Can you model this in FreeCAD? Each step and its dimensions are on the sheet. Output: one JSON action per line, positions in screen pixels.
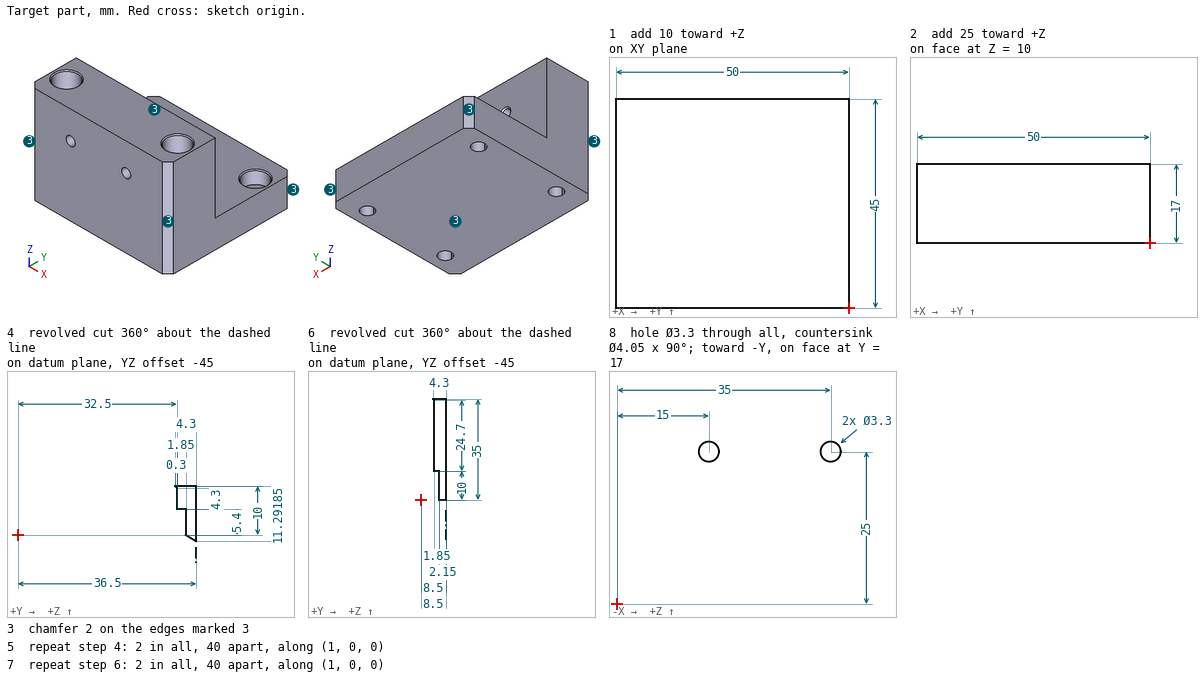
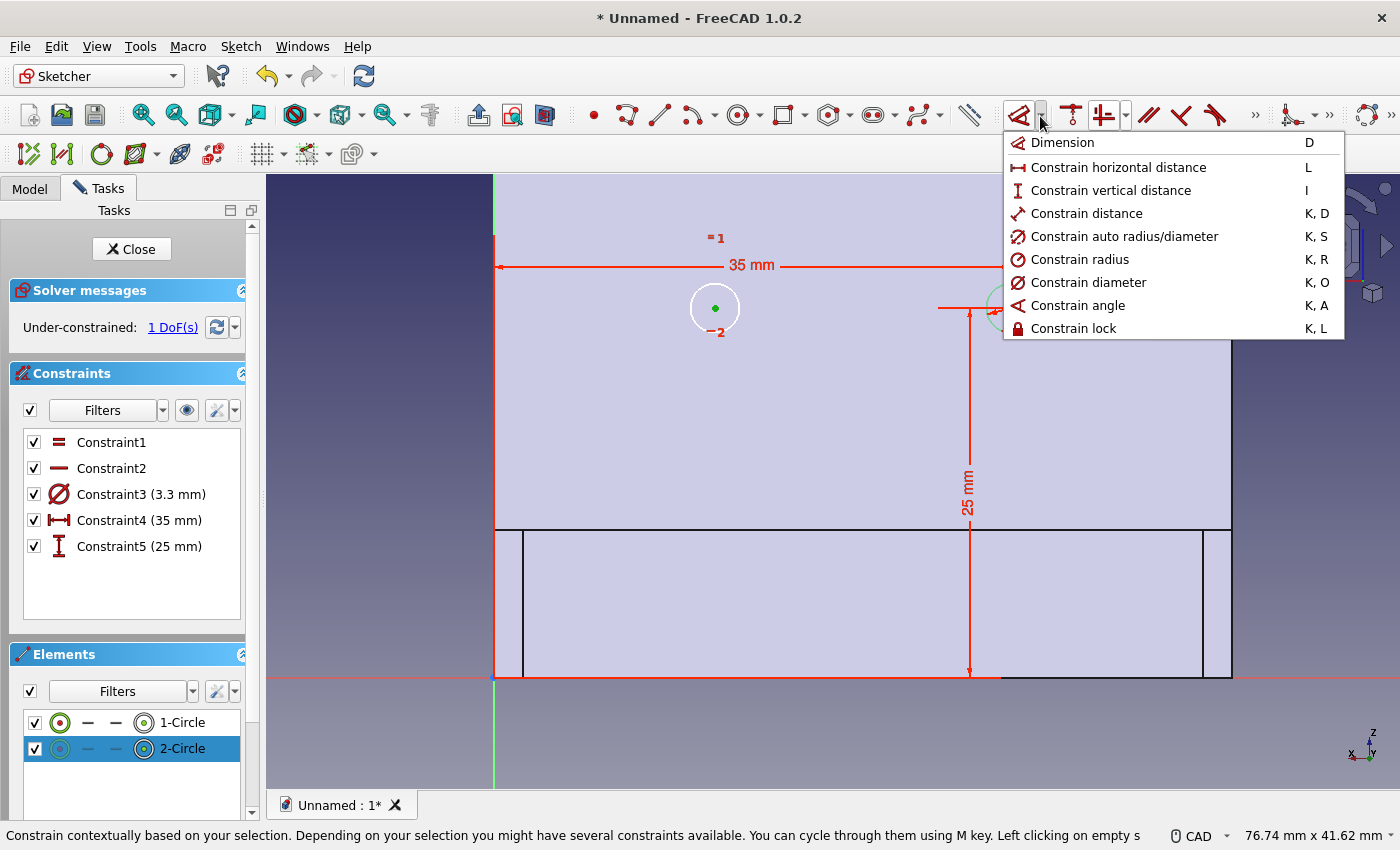
{"action": "left_click", "coordinate": [1174, 168]}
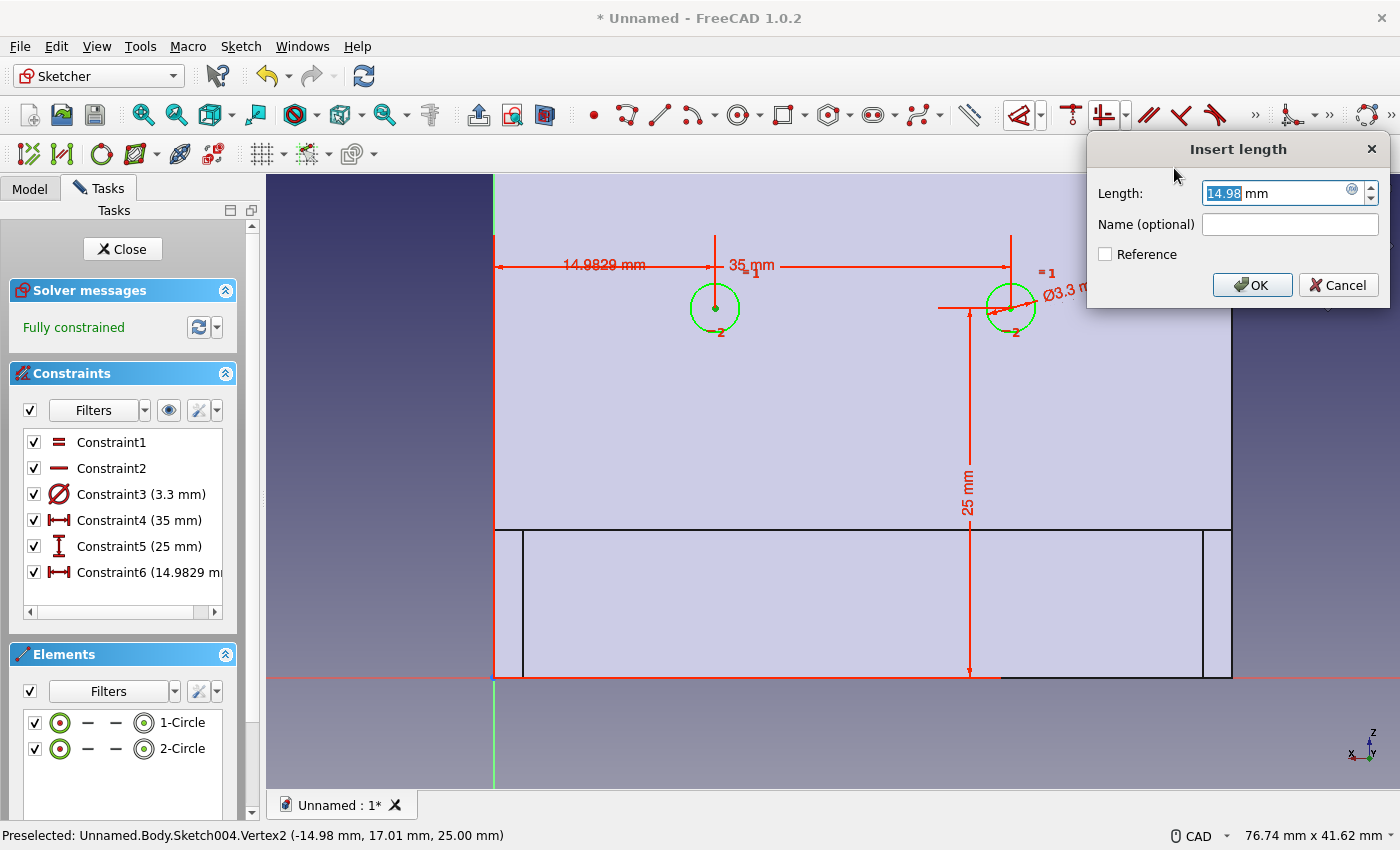
{"action": "type", "text": "15"}
{"action": "key", "text": "Return"}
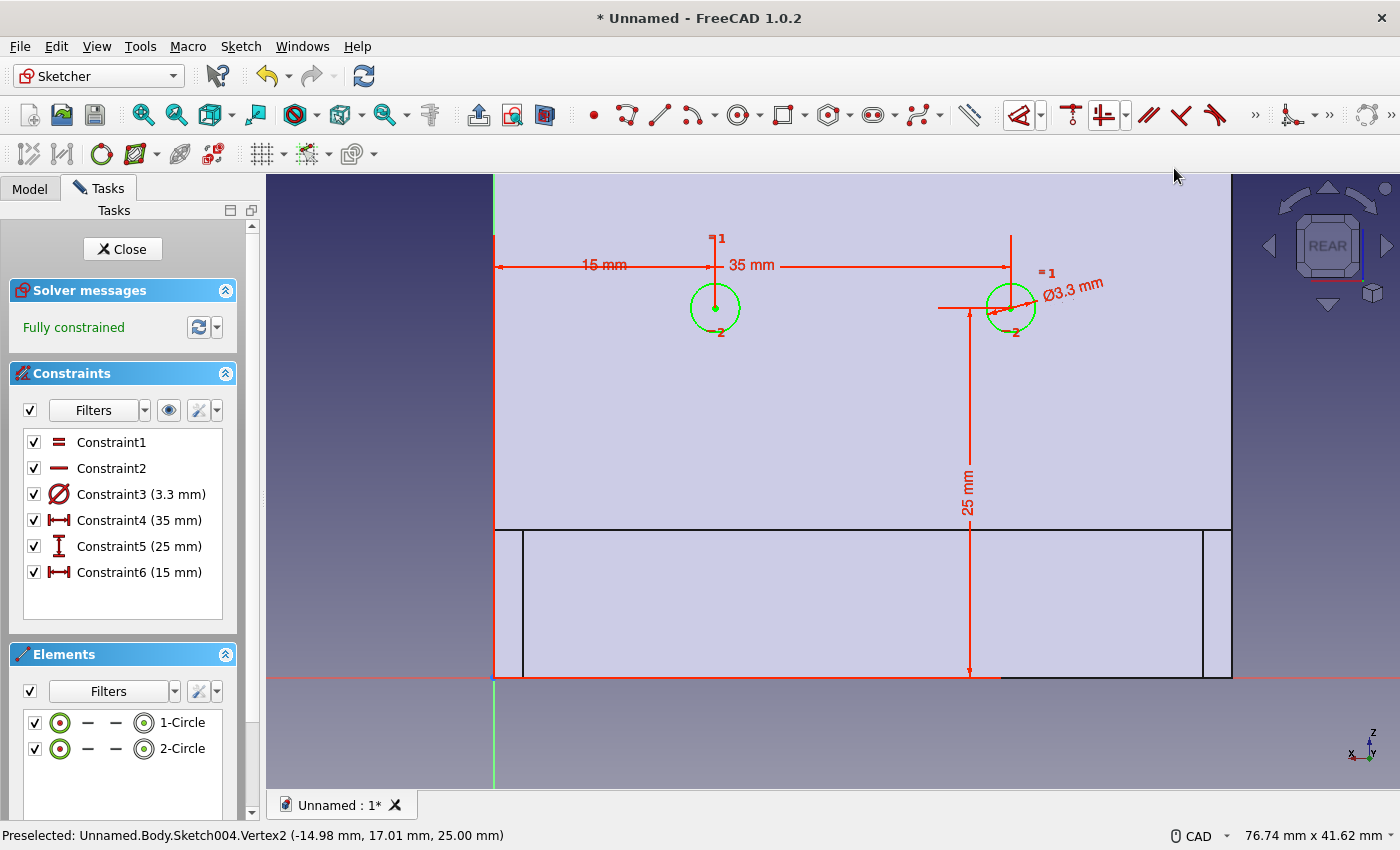
{"action": "left_click", "coordinate": [123, 249]}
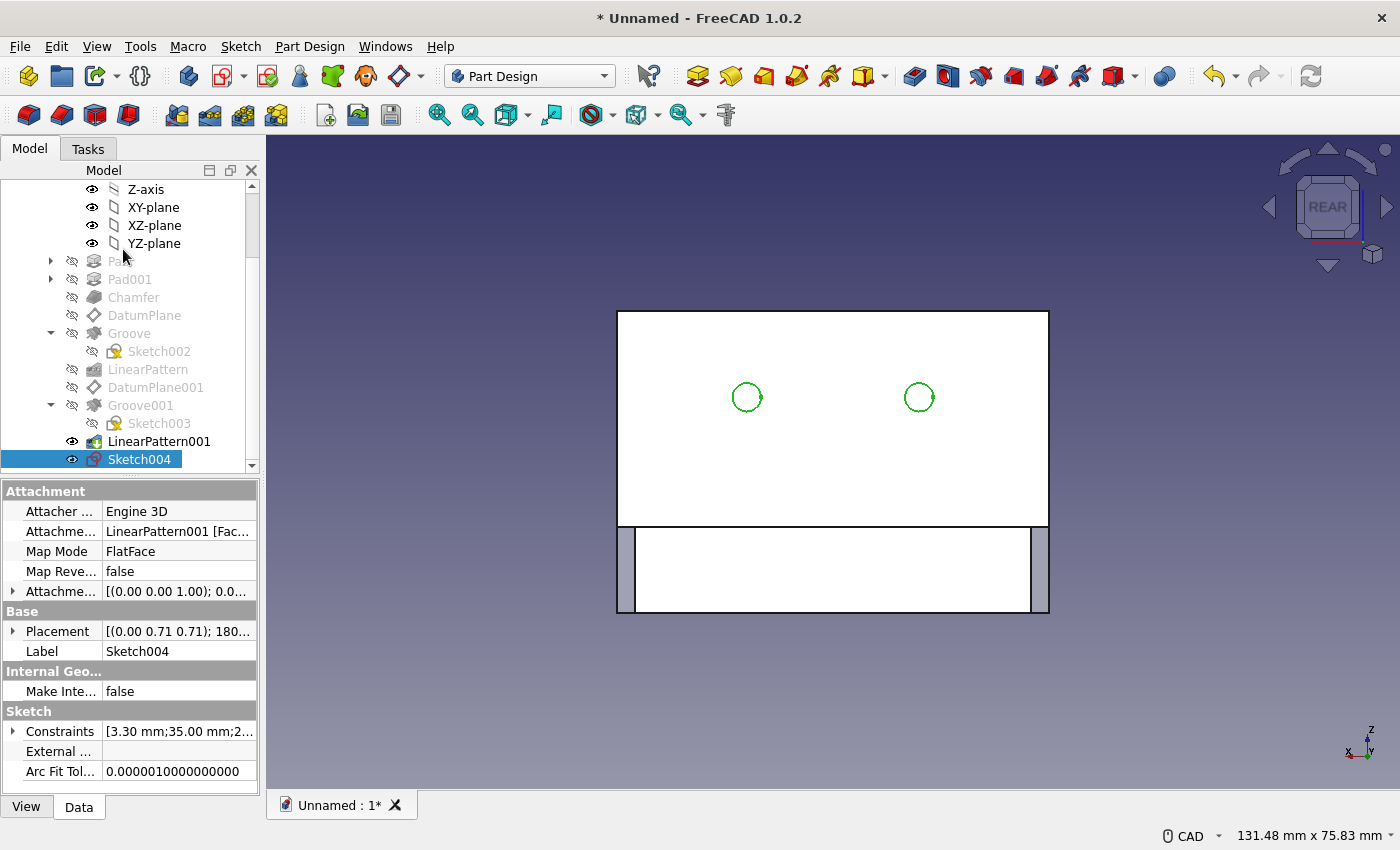
{"action": "left_click", "coordinate": [948, 76]}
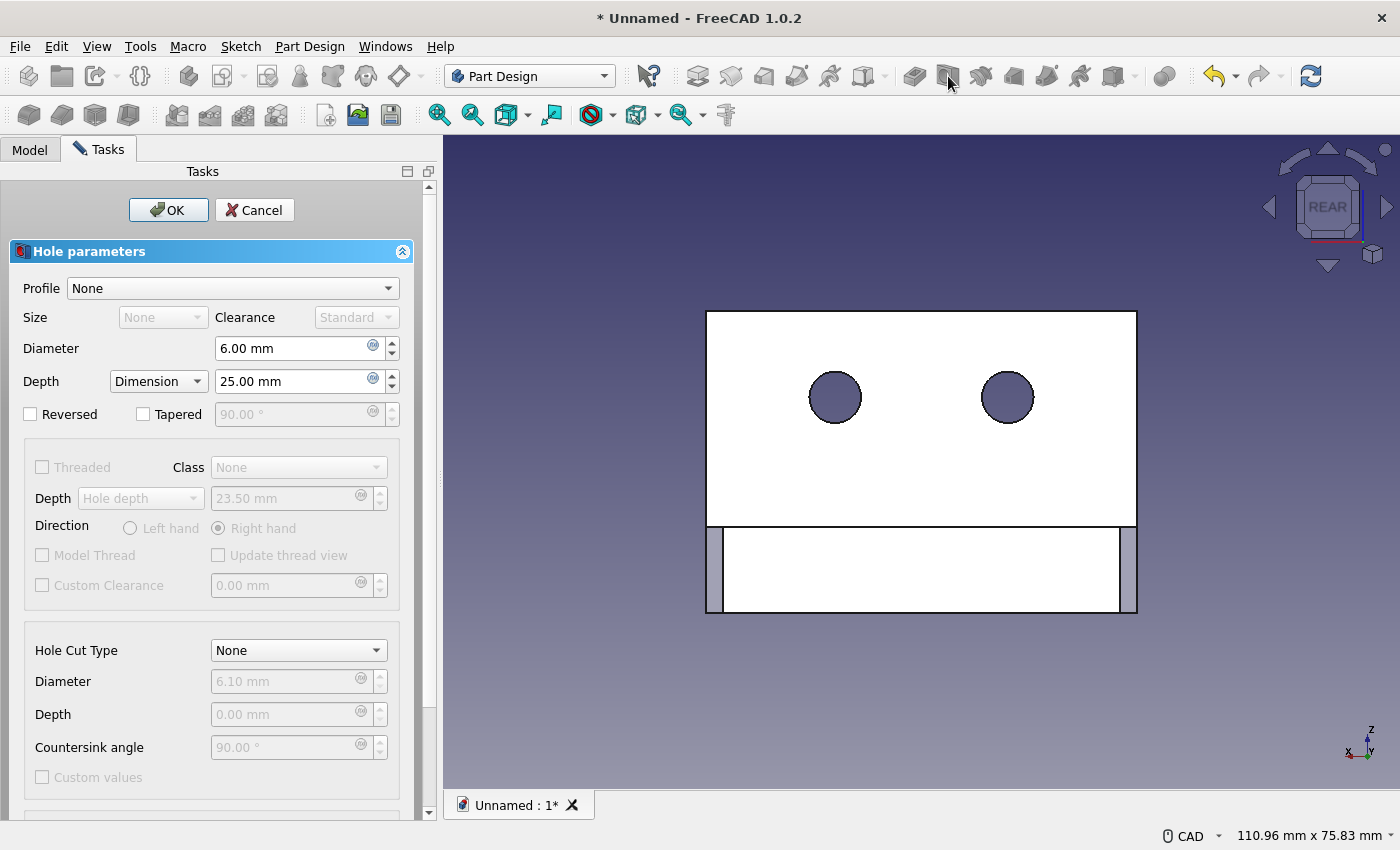
{"action": "triple_click", "coordinate": [300, 348]}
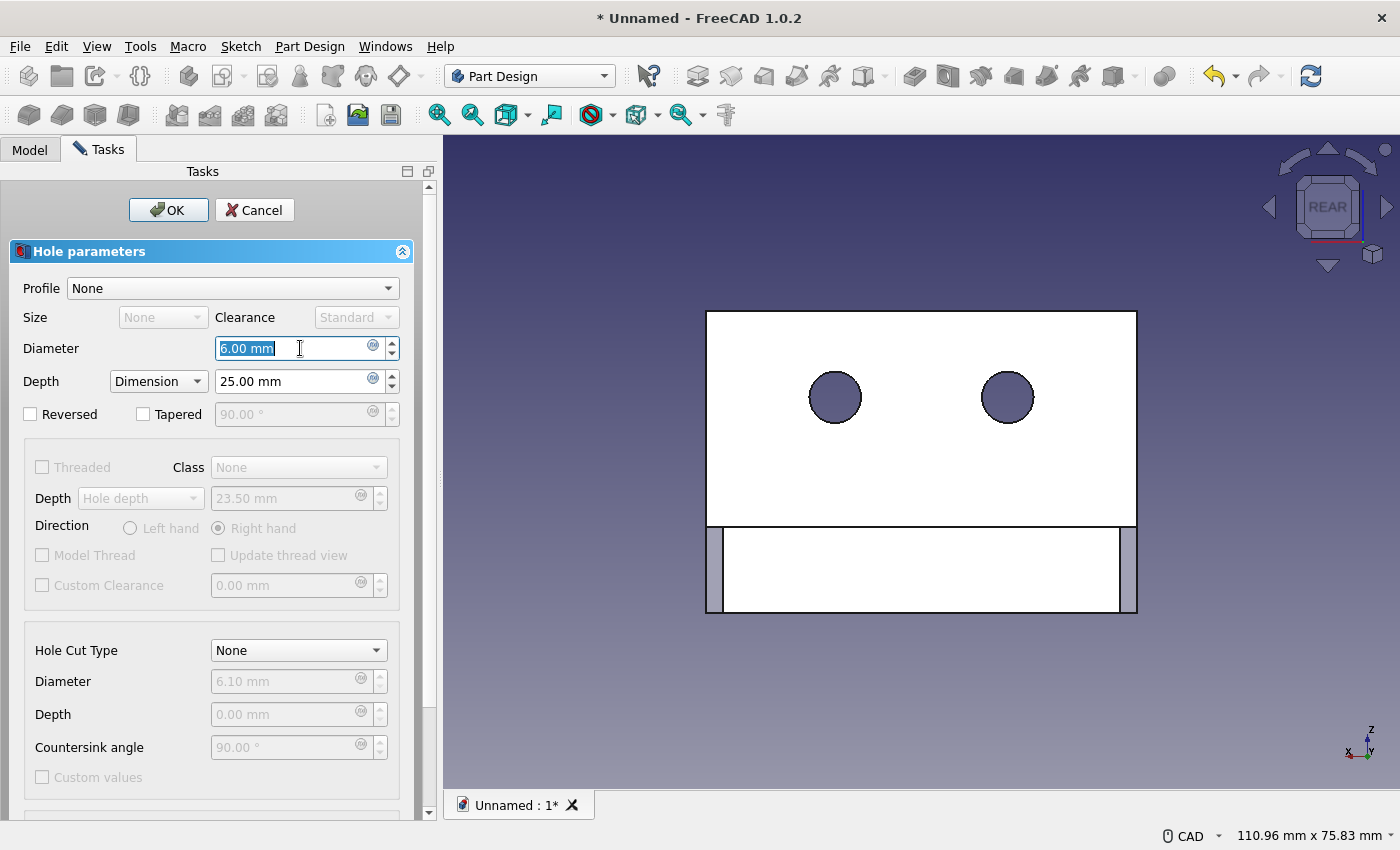
{"action": "type", "text": "3.3"}
{"action": "key", "text": "Tab"}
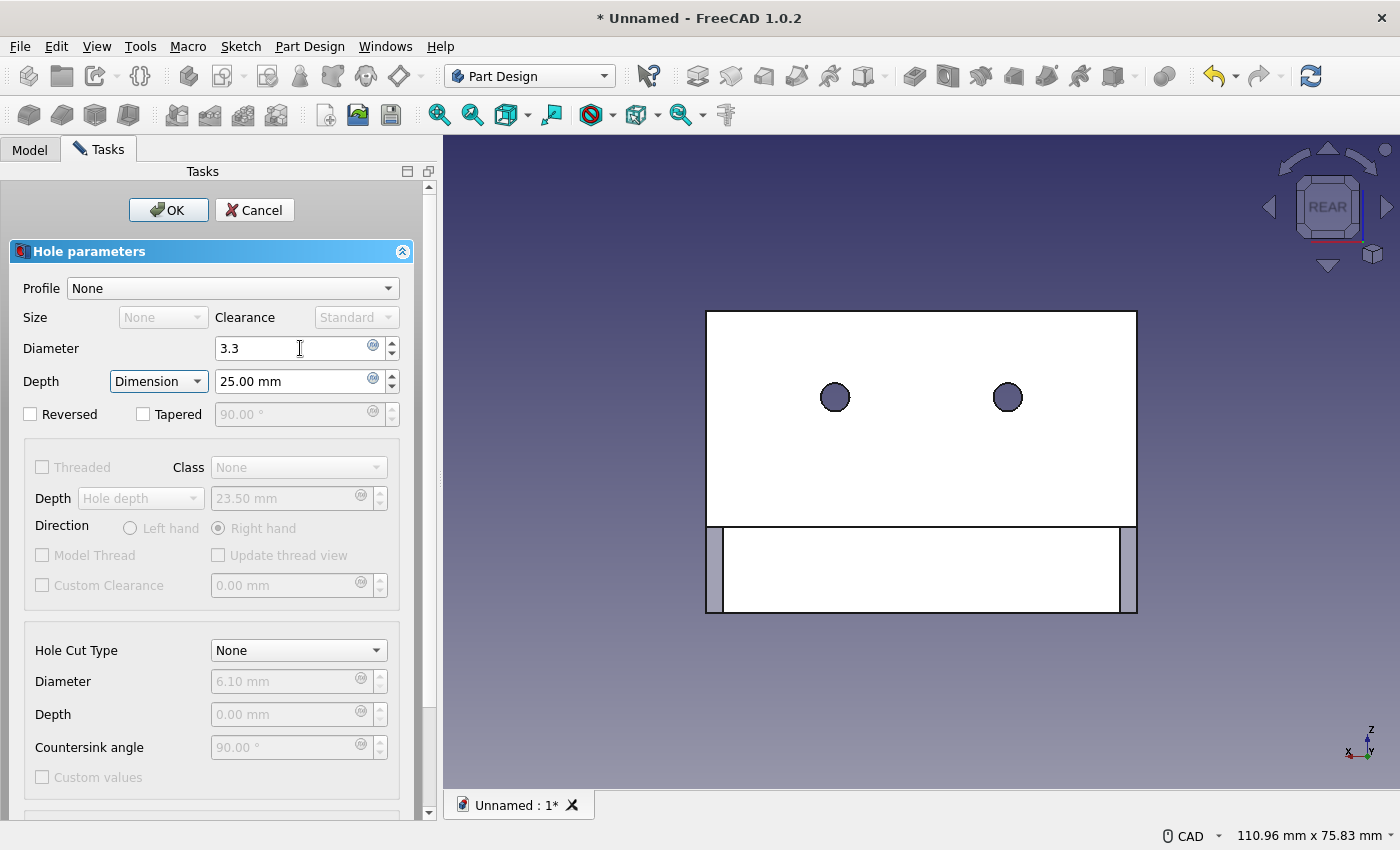
{"action": "left_click", "coordinate": [160, 382]}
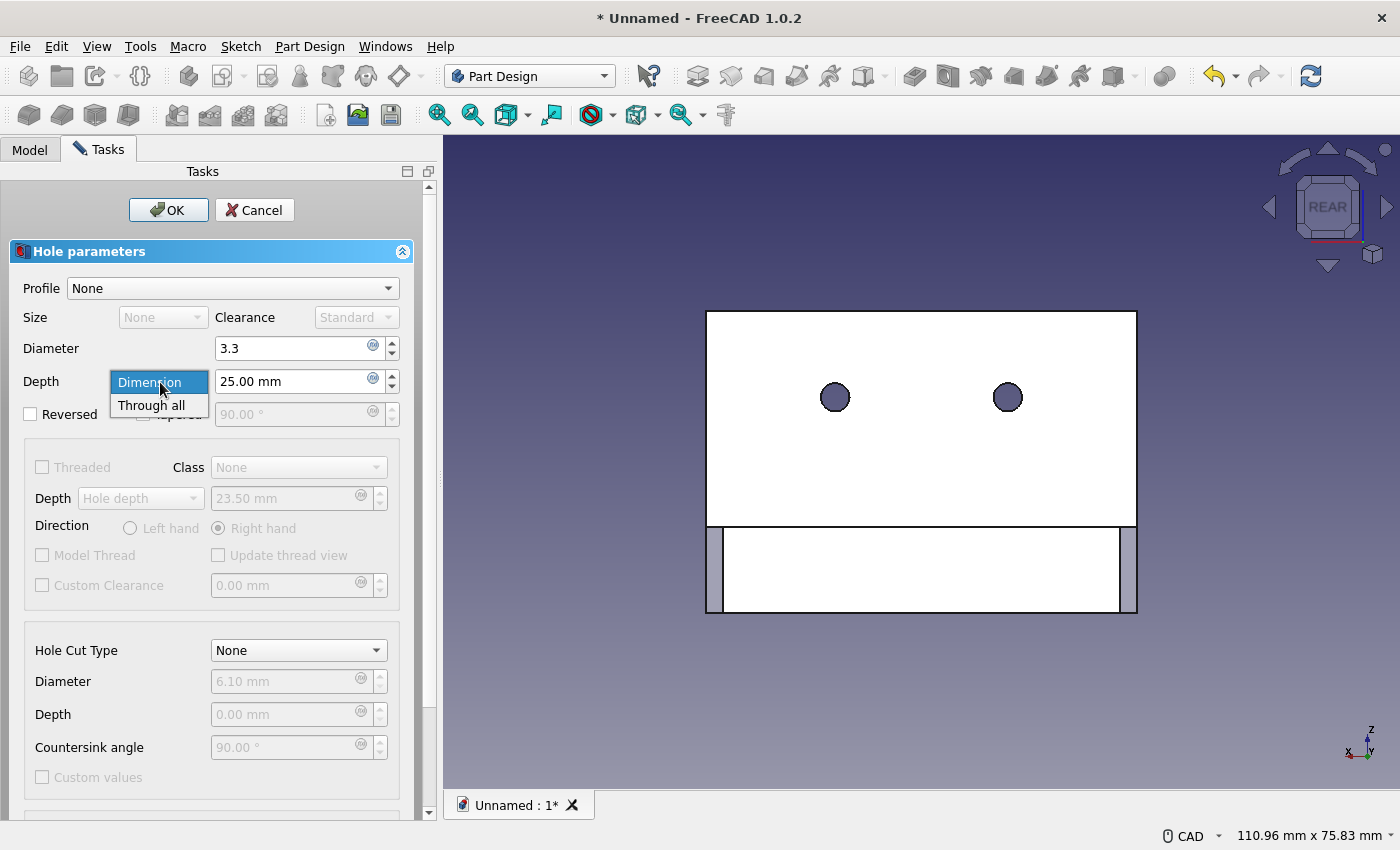
{"action": "left_click", "coordinate": [158, 406]}